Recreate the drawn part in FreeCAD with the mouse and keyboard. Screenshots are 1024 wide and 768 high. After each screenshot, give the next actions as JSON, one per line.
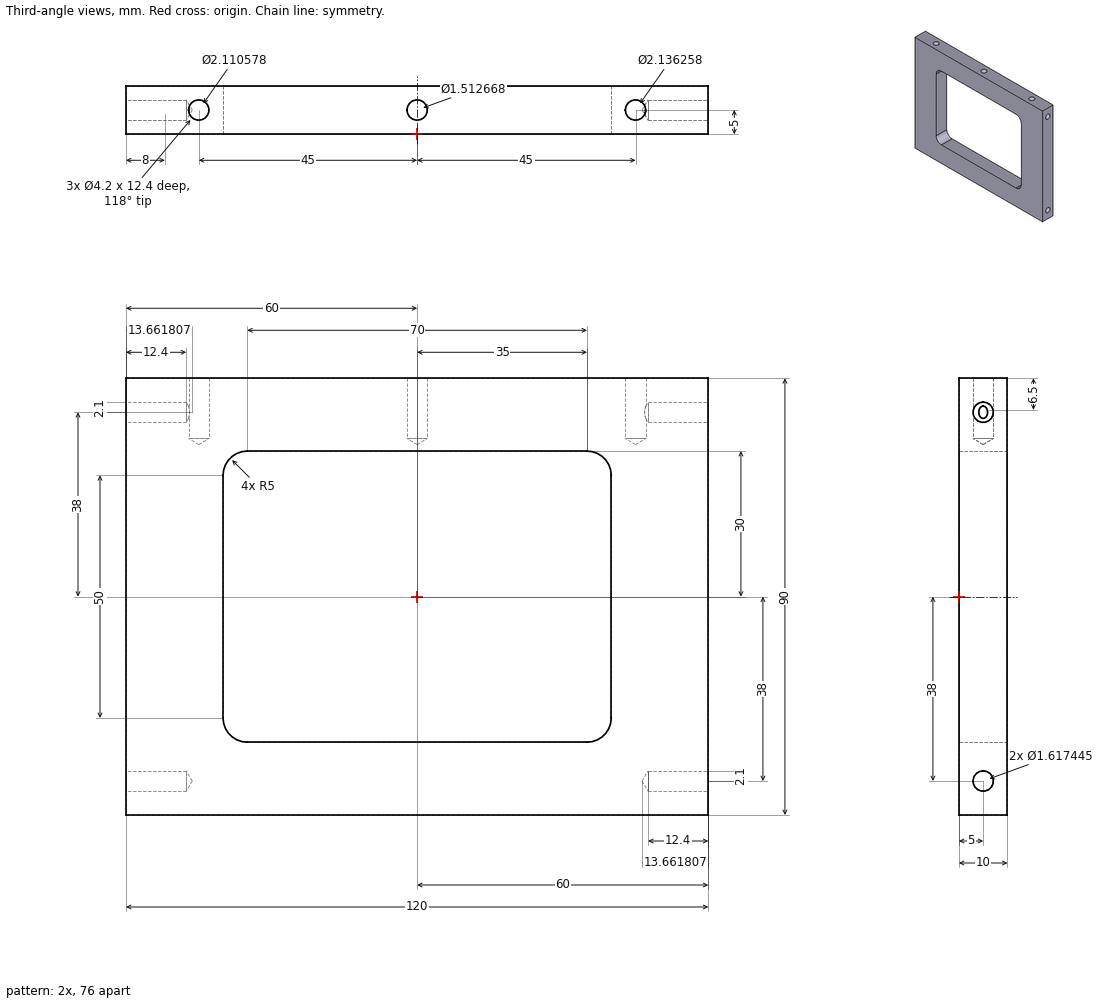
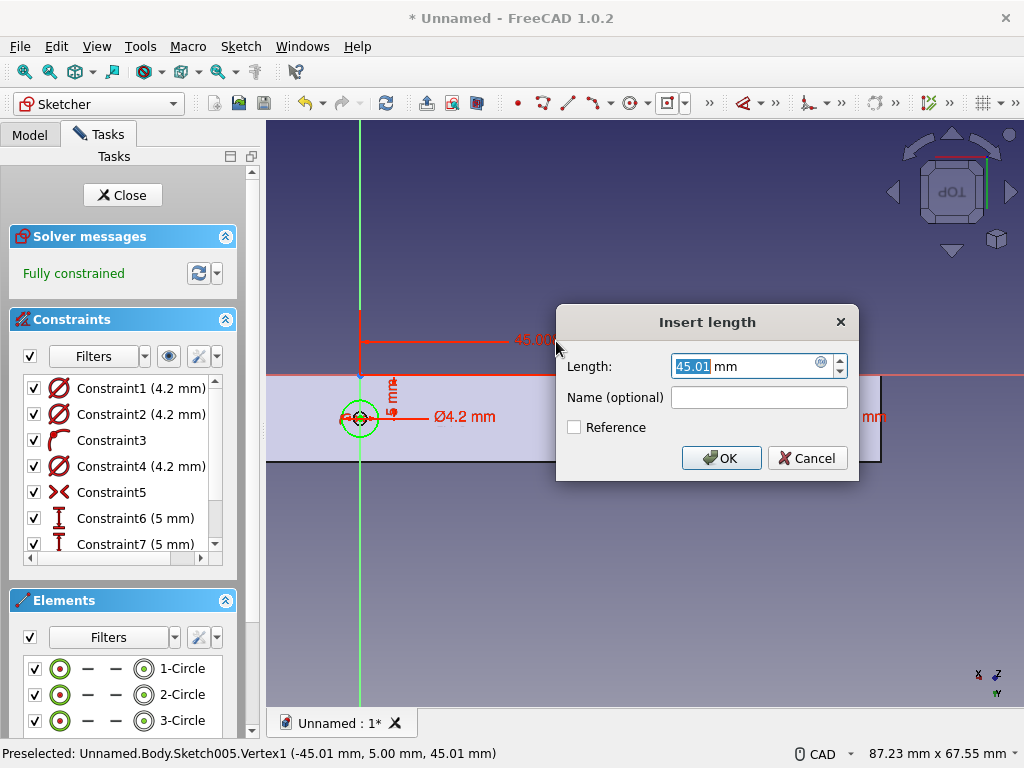
{"action": "type", "text": "45"}
{"action": "key", "text": "Return"}
{"action": "key", "text": "Escape"}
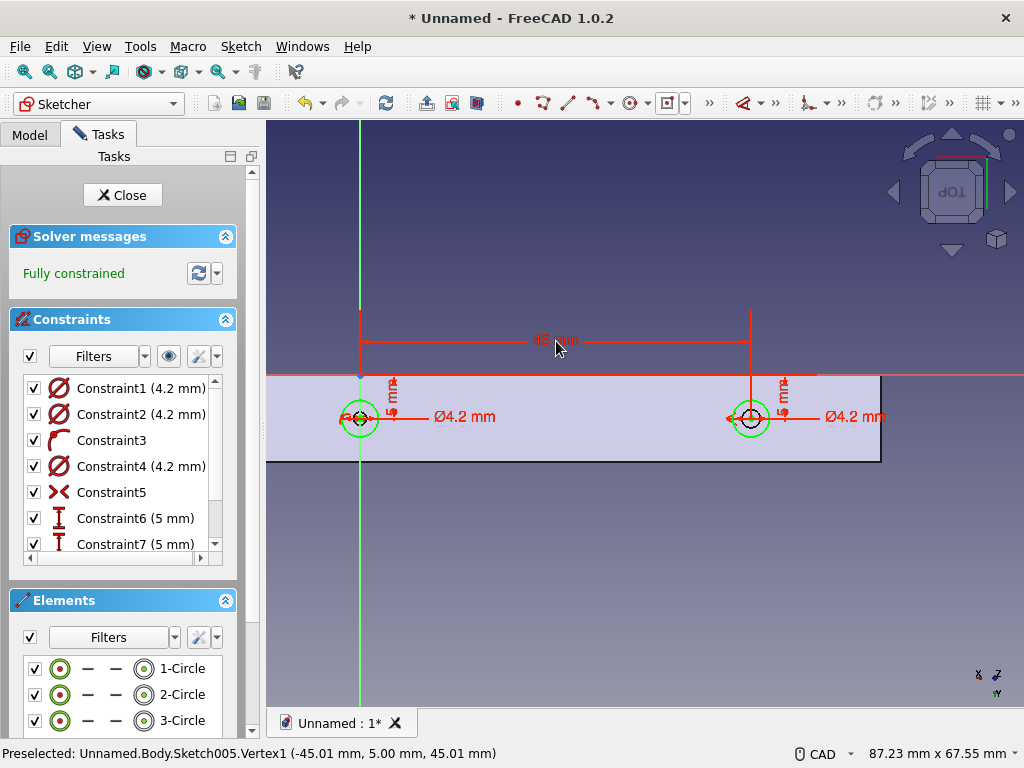
{"action": "left_click", "coordinate": [123, 195]}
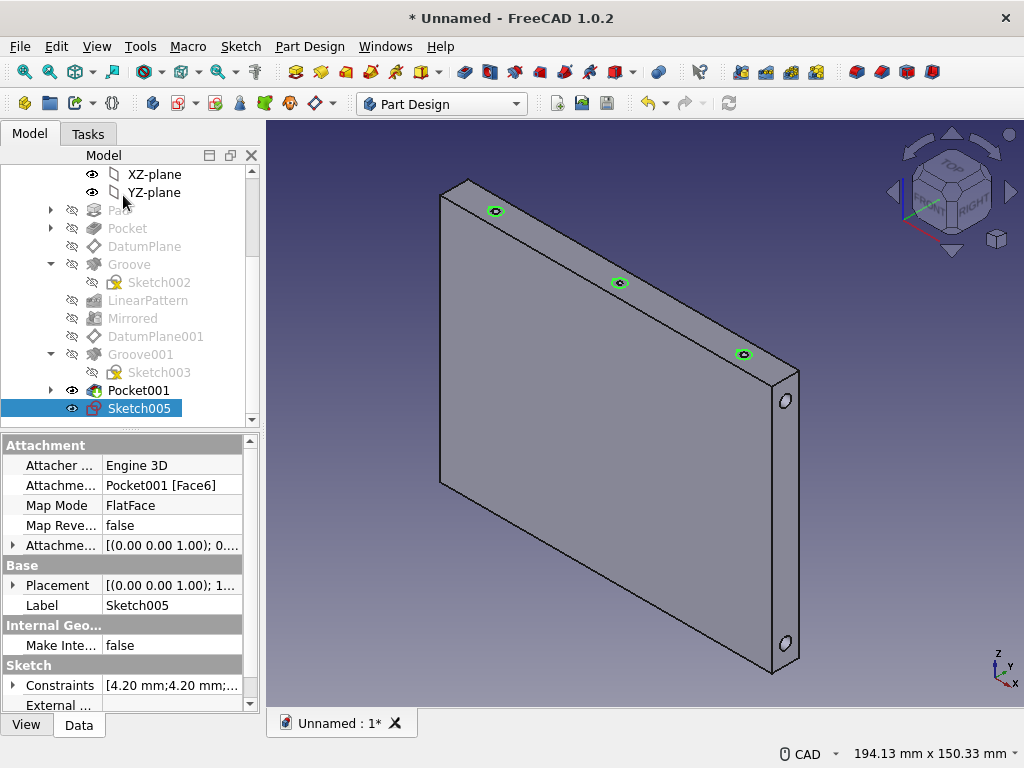
{"action": "left_click", "coordinate": [490, 72]}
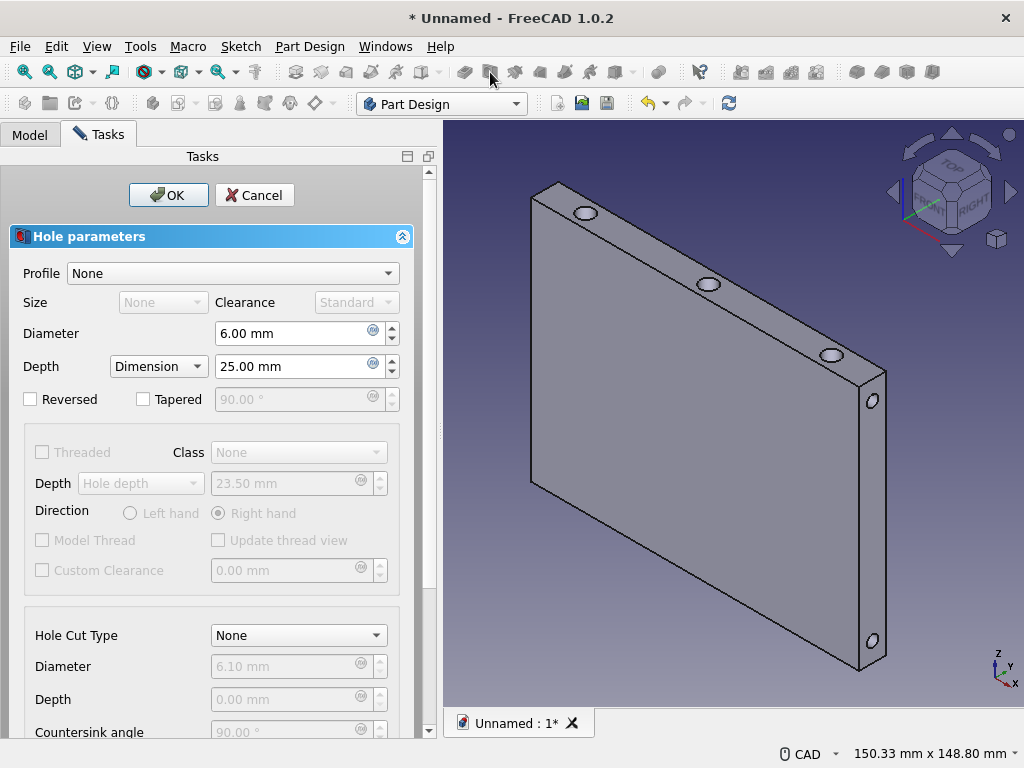
{"action": "triple_click", "coordinate": [300, 334]}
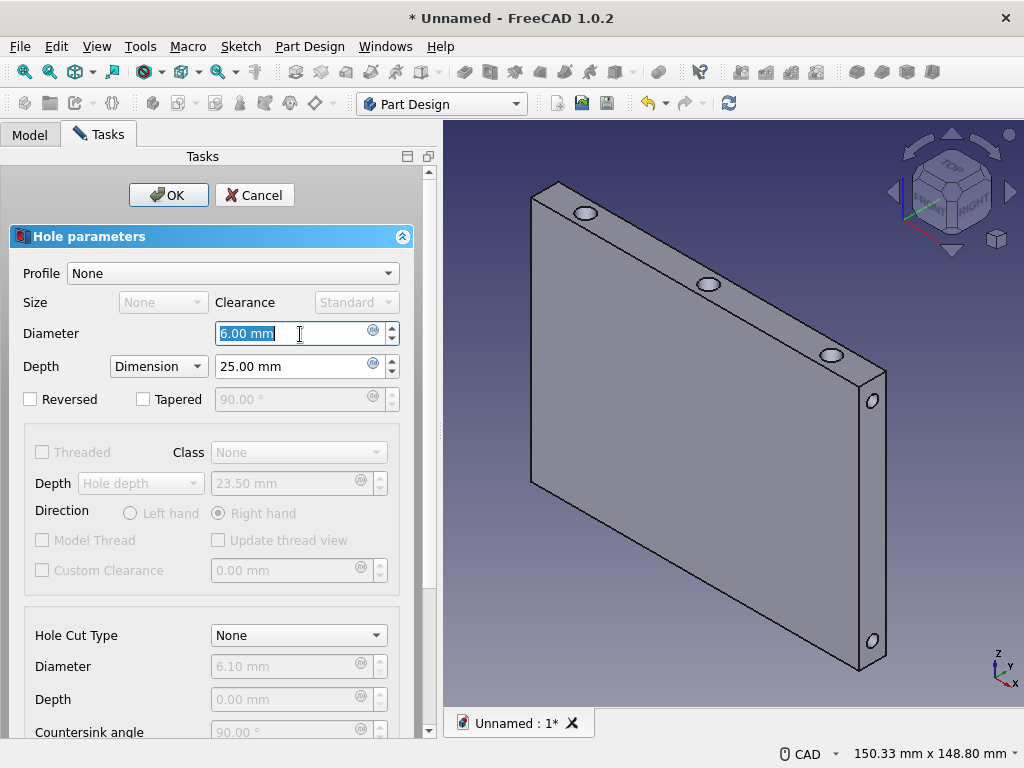
{"action": "type", "text": "4.2"}
{"action": "key", "text": "Tab"}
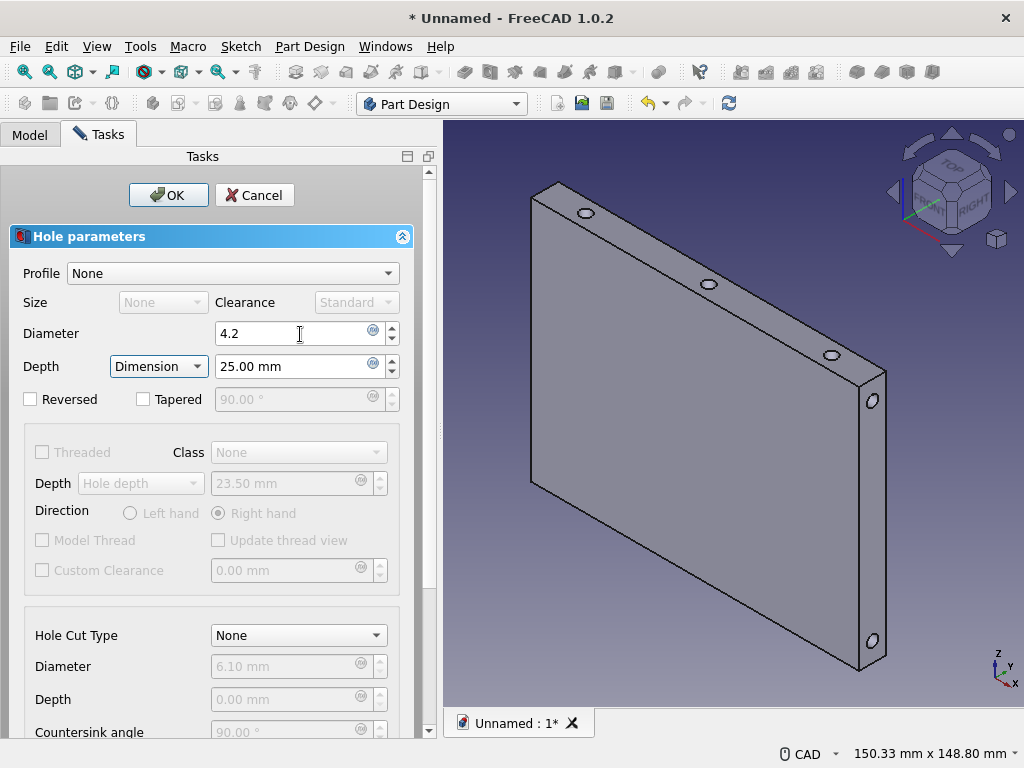
{"action": "triple_click", "coordinate": [300, 366]}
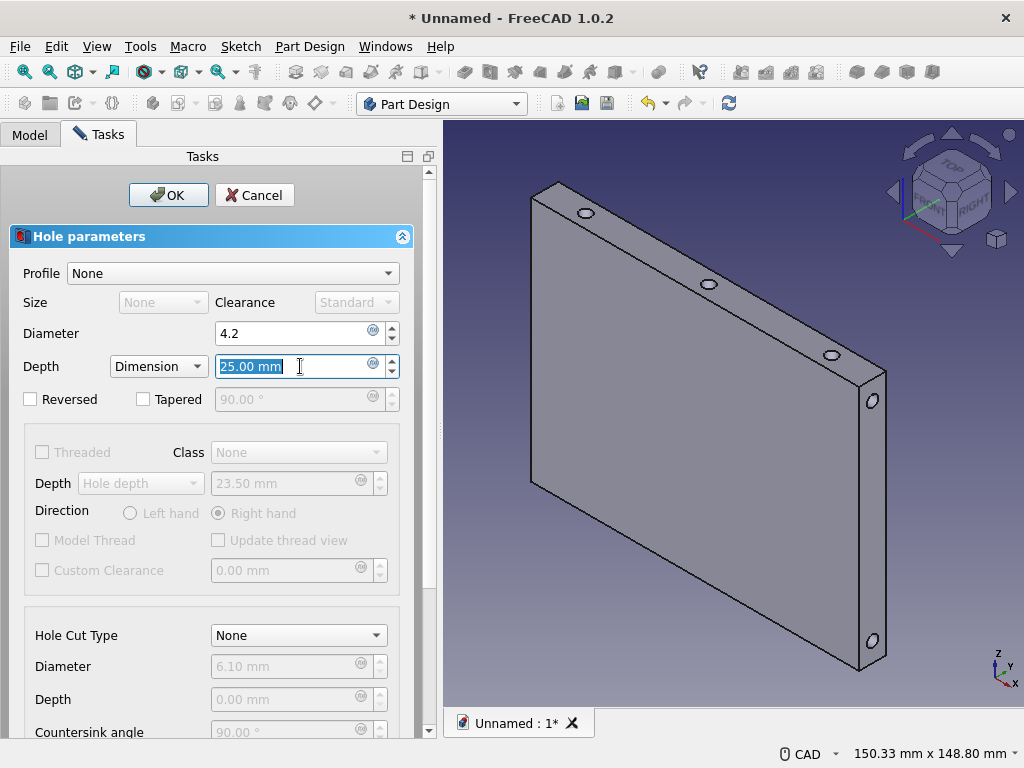
{"action": "type", "text": "12.4"}
{"action": "key", "text": "Tab"}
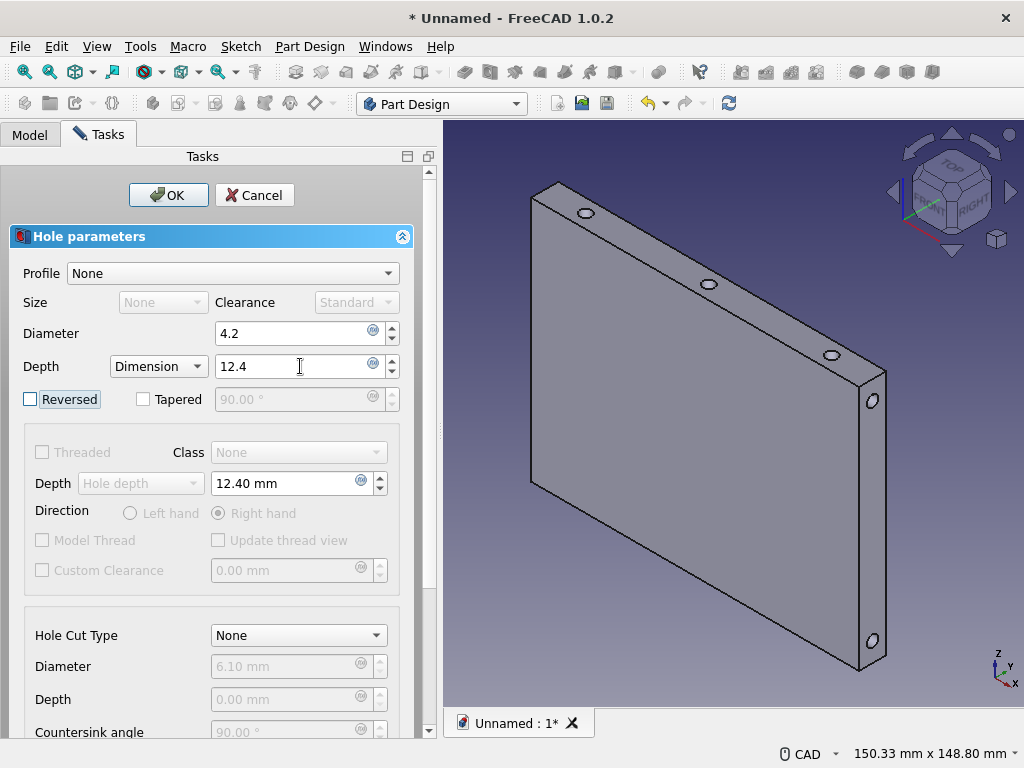
{"action": "left_click", "coordinate": [169, 195]}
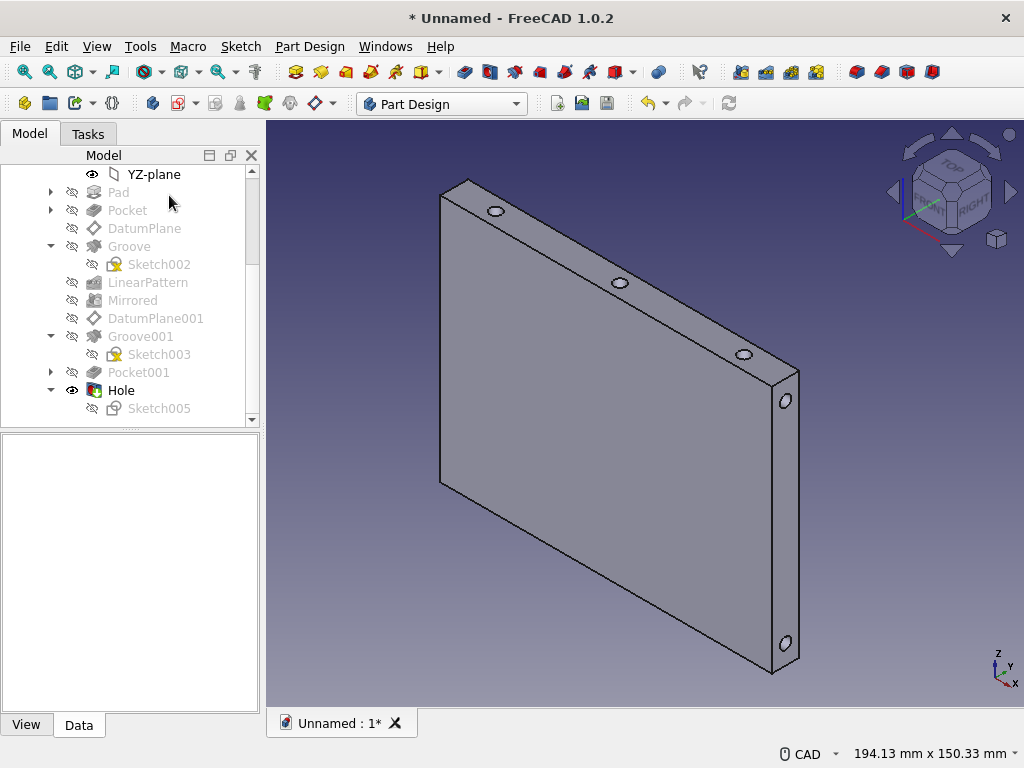
{"action": "left_click", "coordinate": [606, 434]}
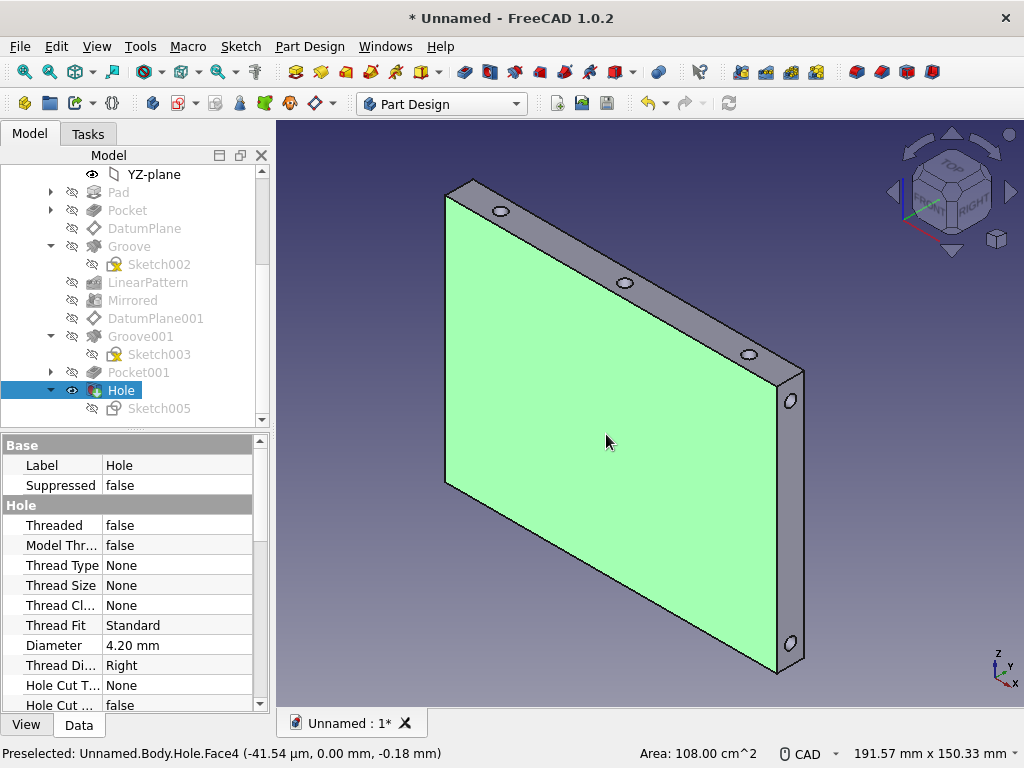
{"action": "left_click", "coordinate": [178, 104]}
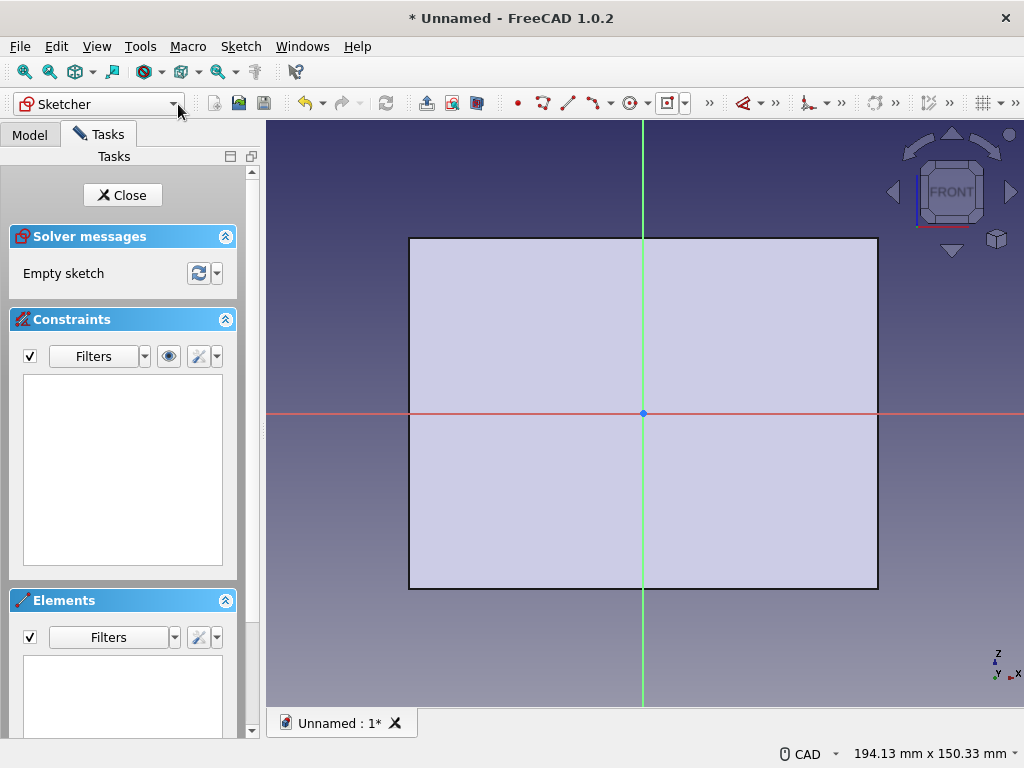
{"action": "left_click", "coordinate": [568, 104]}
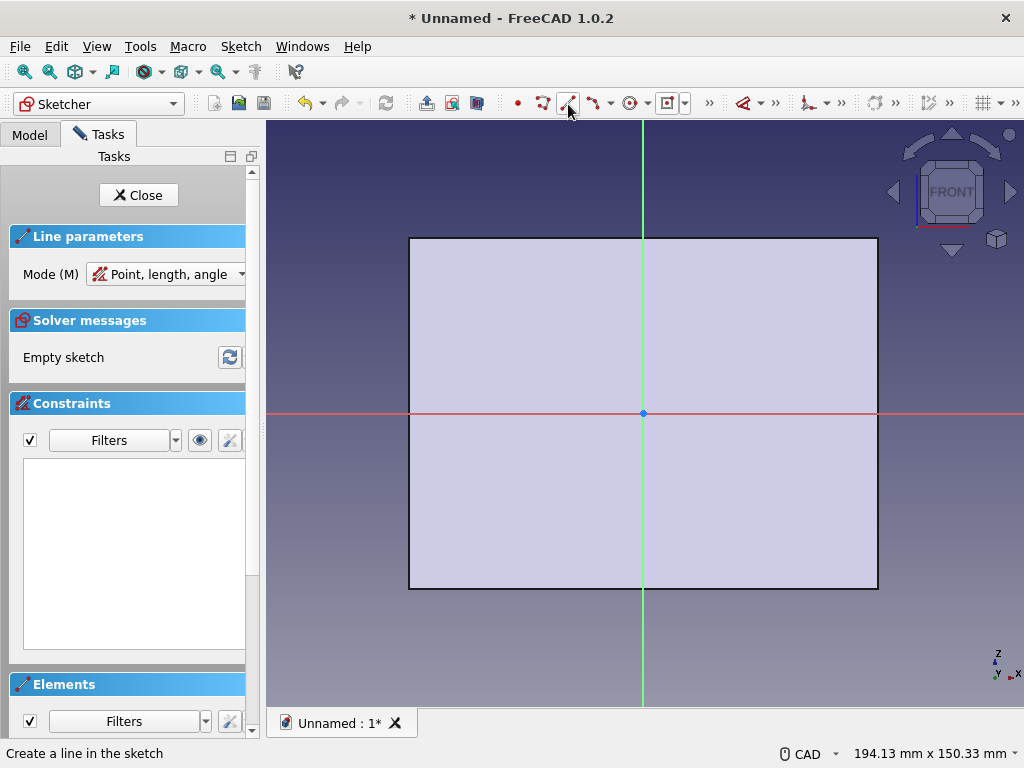
{"action": "left_click", "coordinate": [780, 296]}
{"action": "left_click", "coordinate": [507, 296]}